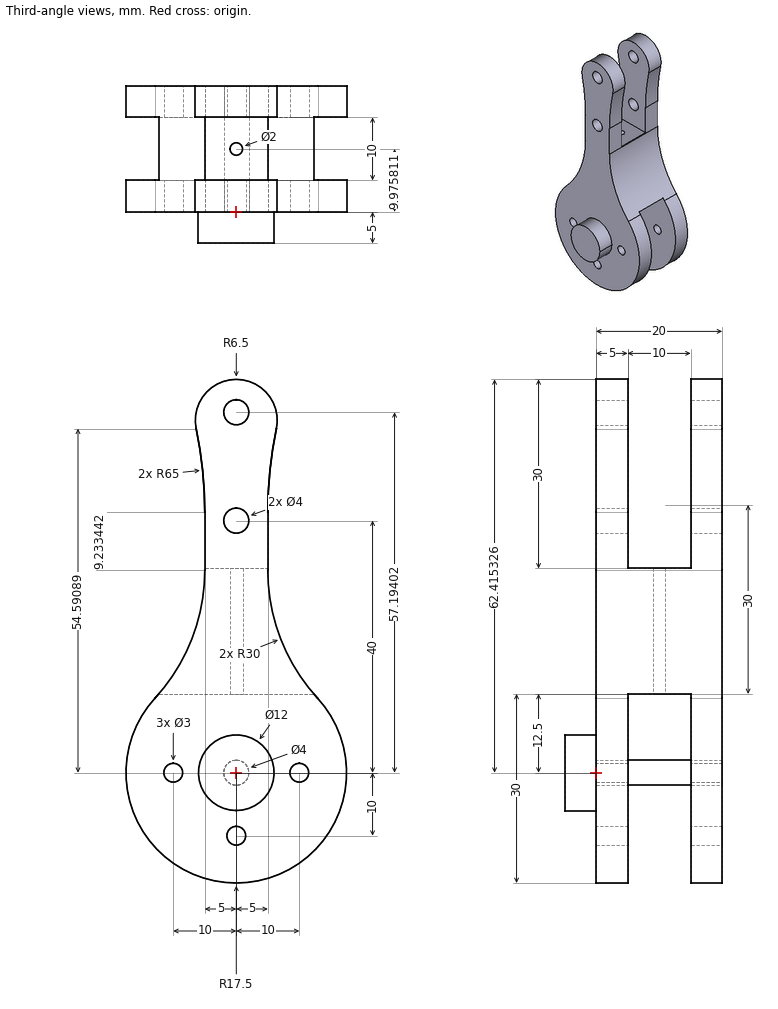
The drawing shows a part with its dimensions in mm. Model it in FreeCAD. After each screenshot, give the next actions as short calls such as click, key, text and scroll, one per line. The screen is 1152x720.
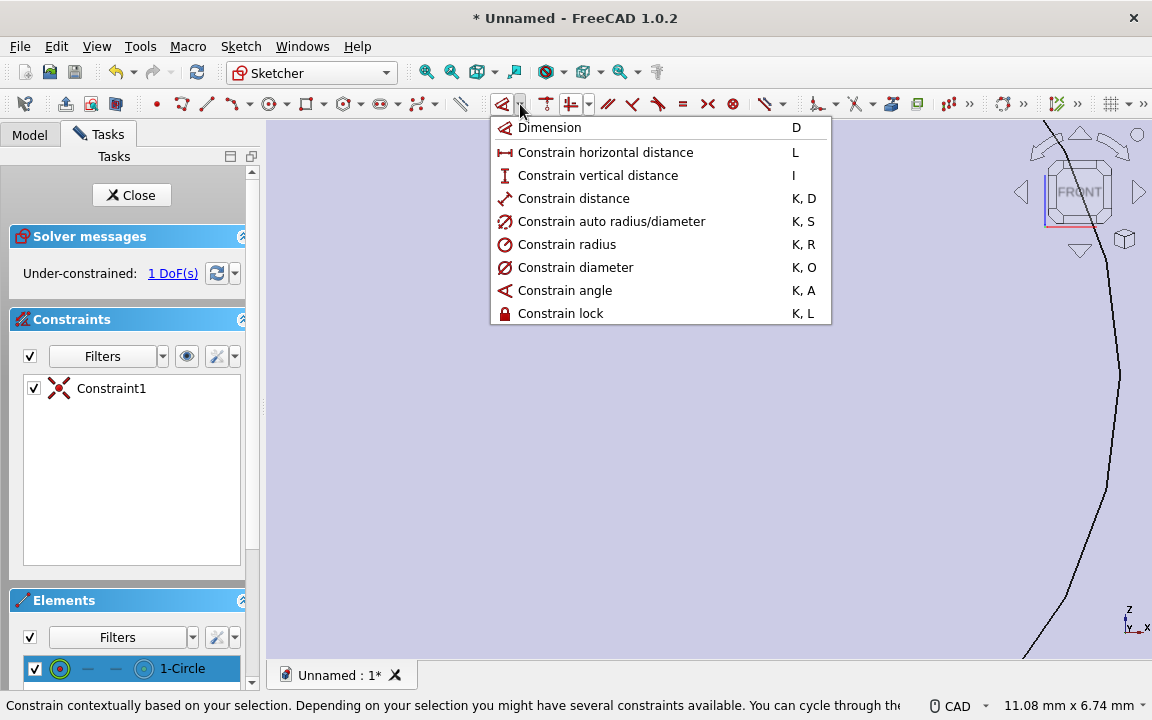
click(661, 268)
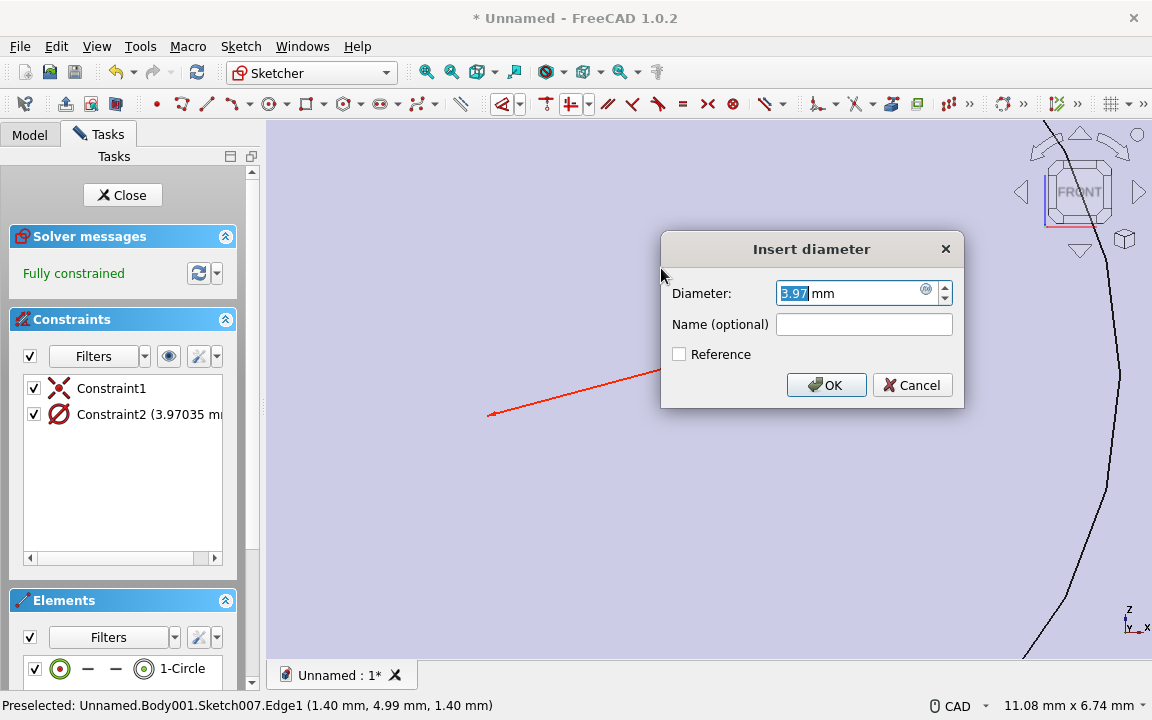
text(4)
key(Return)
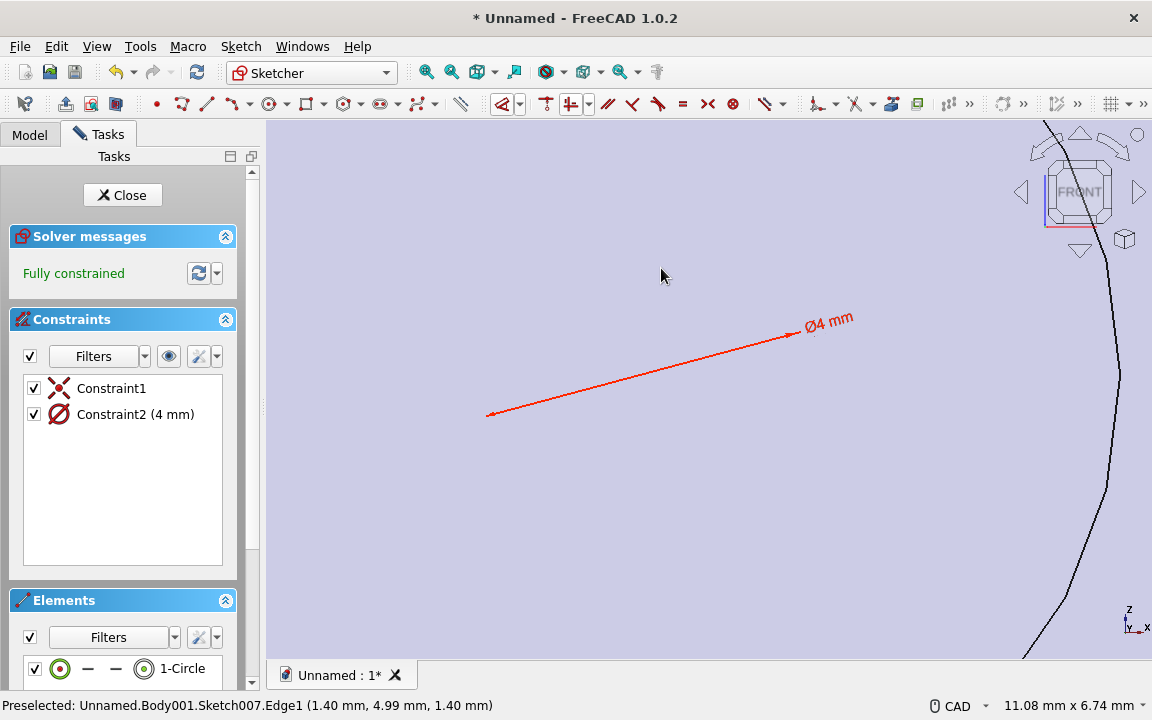
click(123, 195)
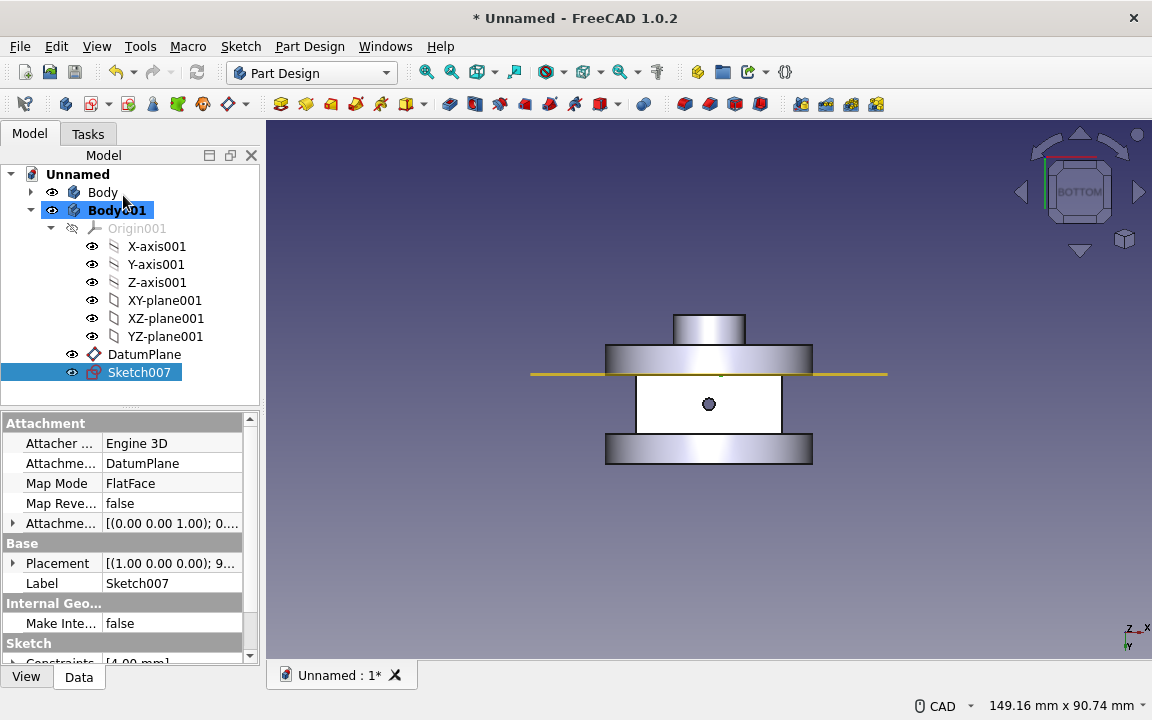
click(281, 104)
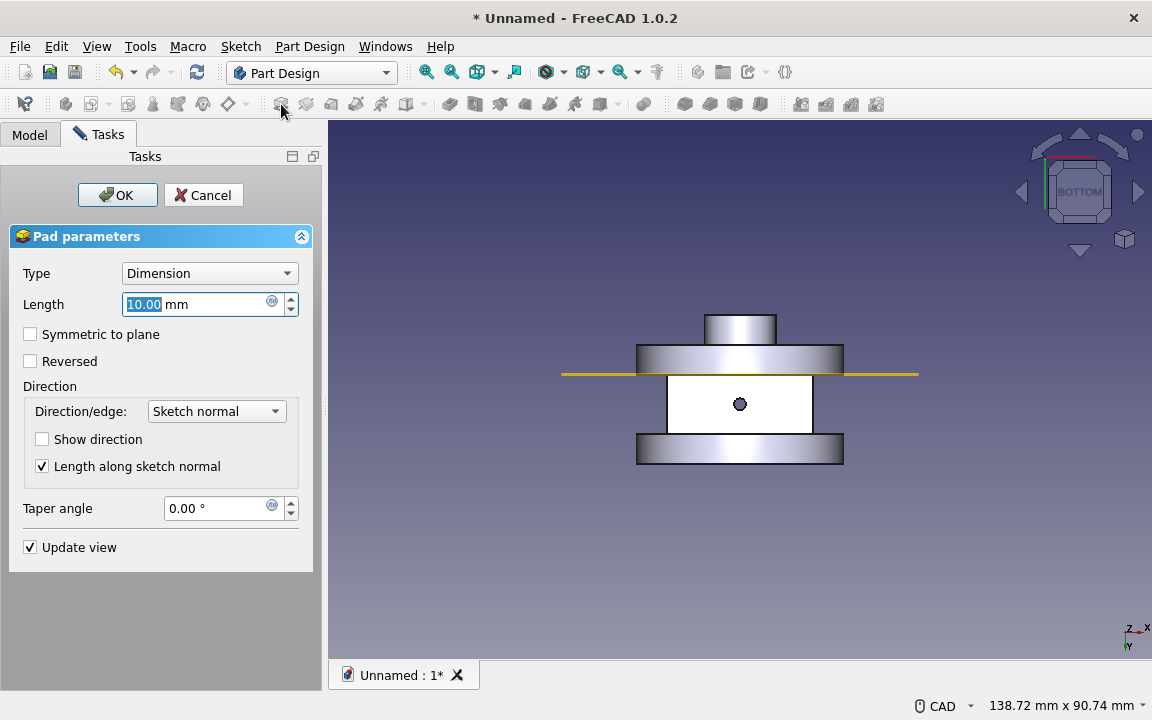
text(10)
key(Tab)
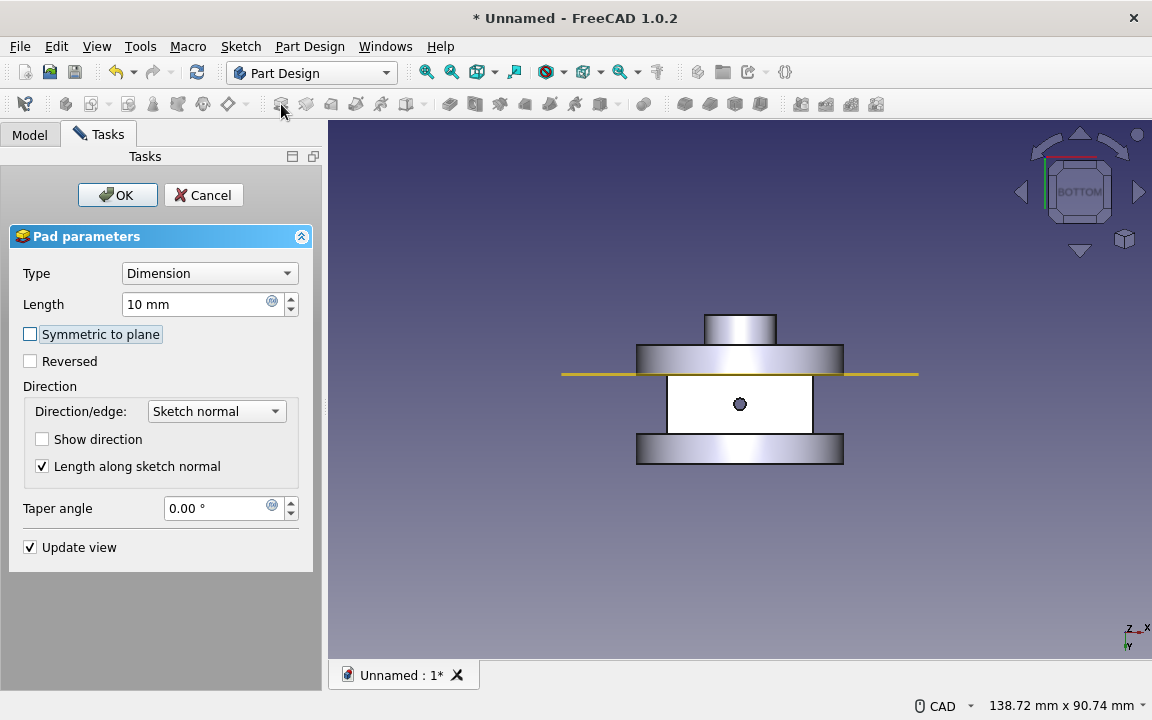
click(31, 361)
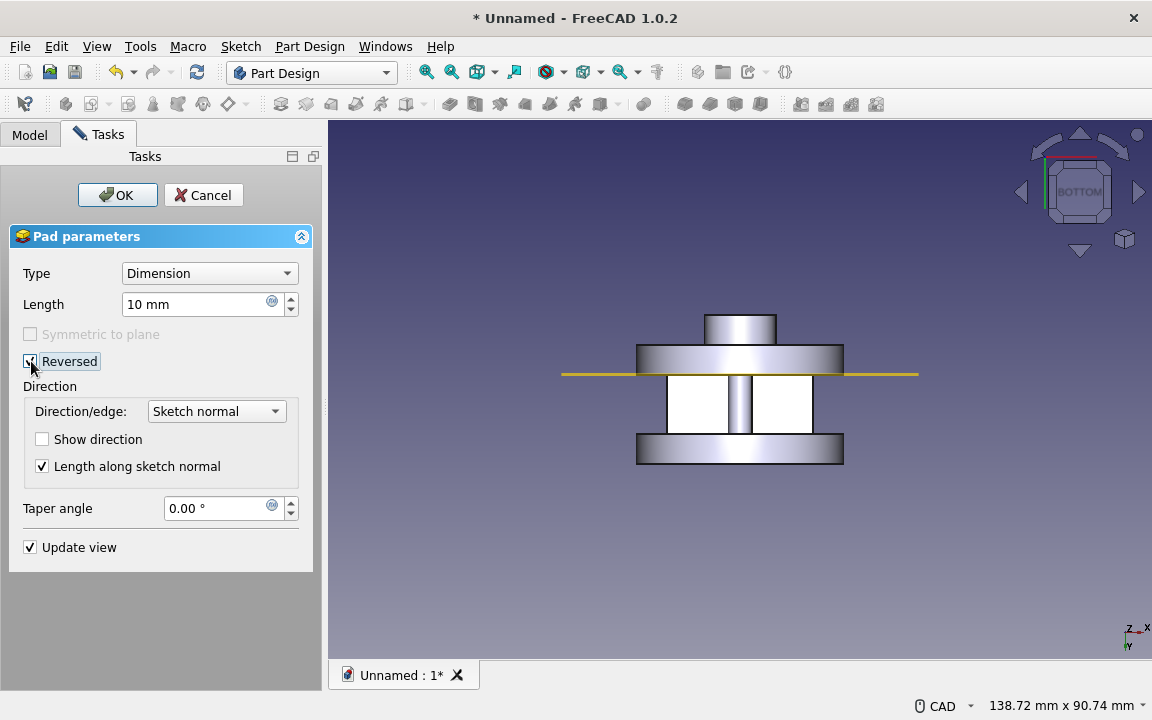
click(118, 195)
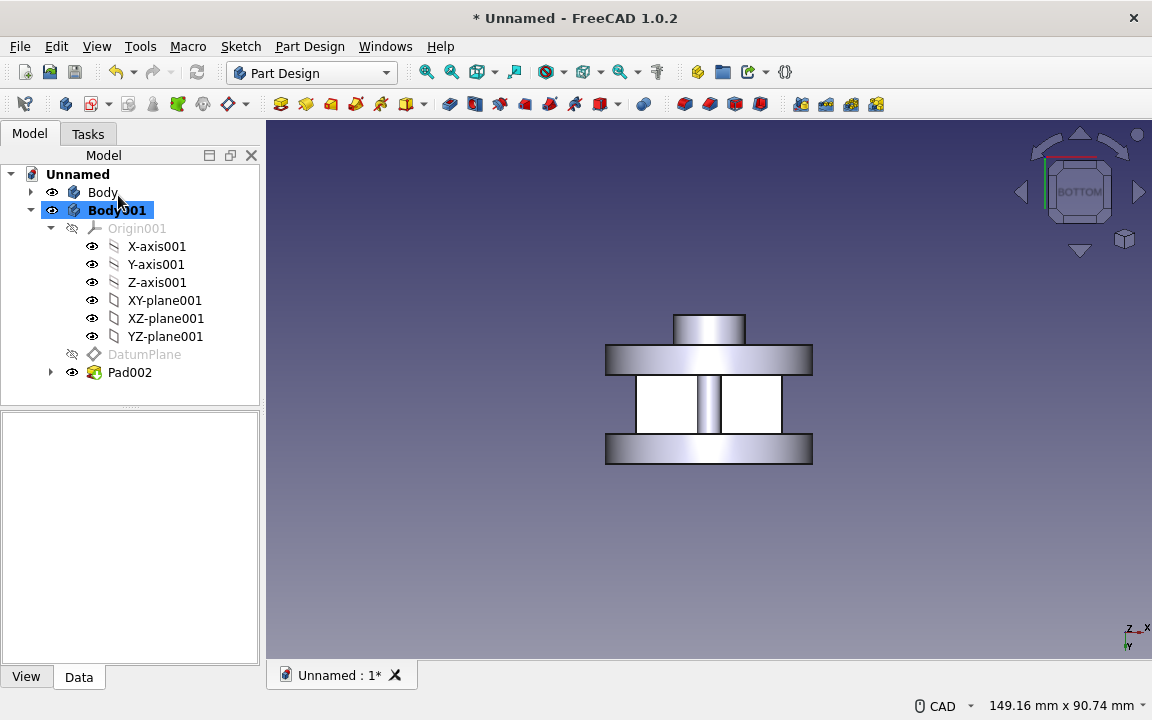
key(0)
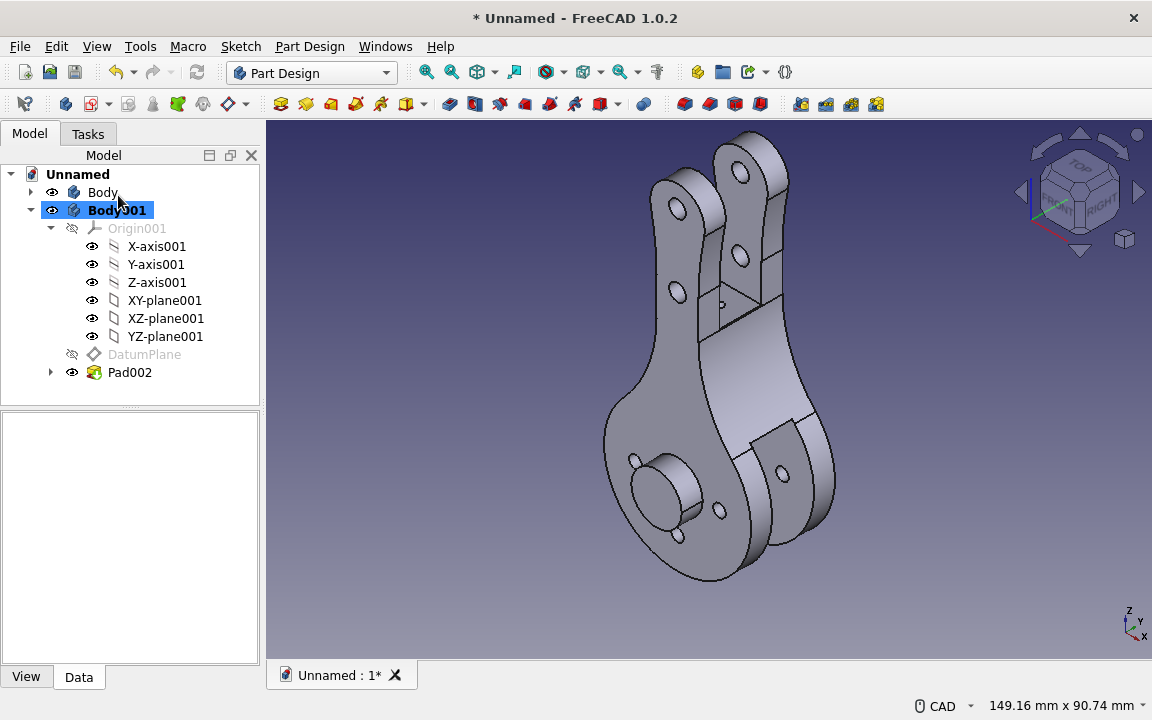
click(427, 72)